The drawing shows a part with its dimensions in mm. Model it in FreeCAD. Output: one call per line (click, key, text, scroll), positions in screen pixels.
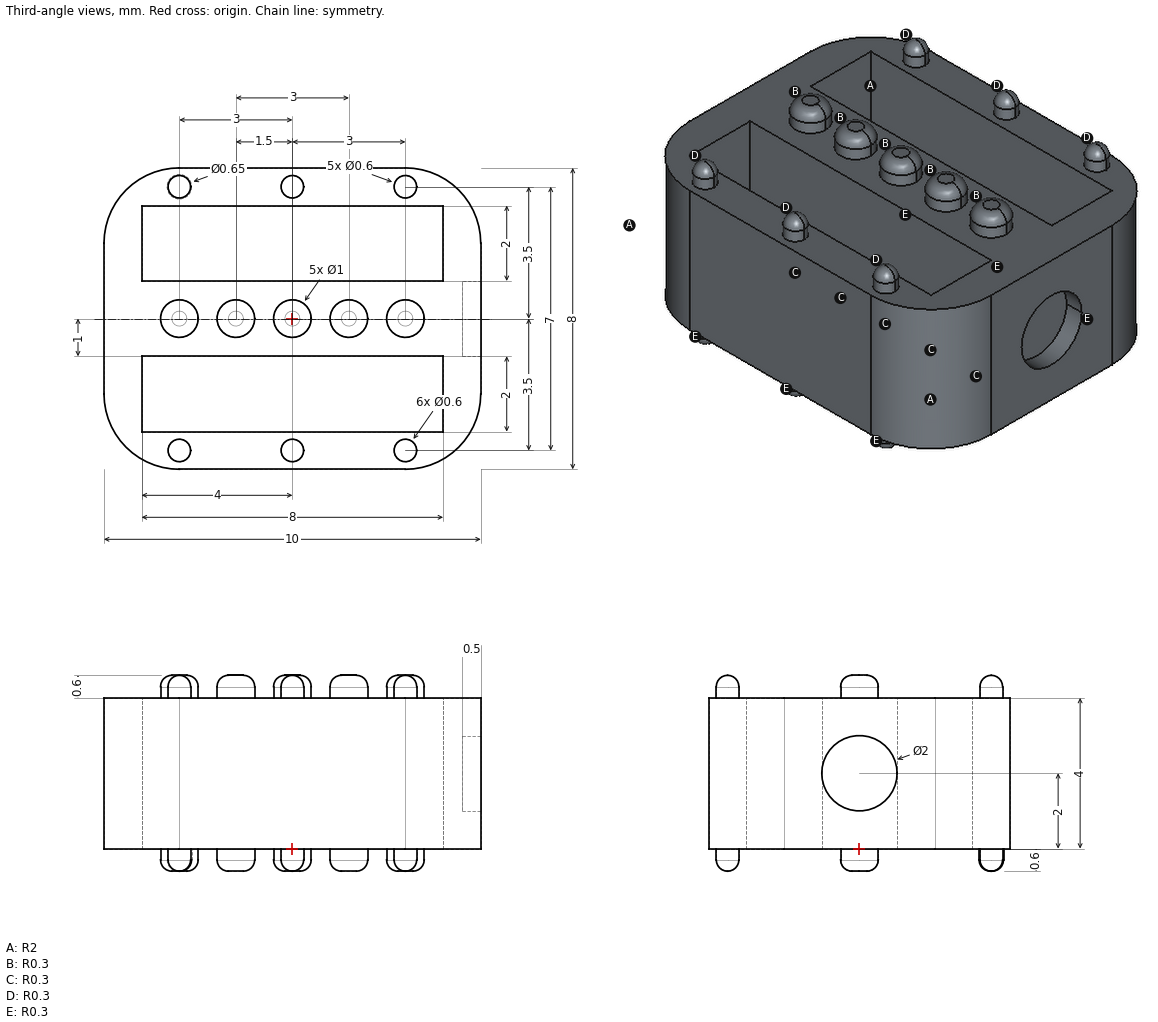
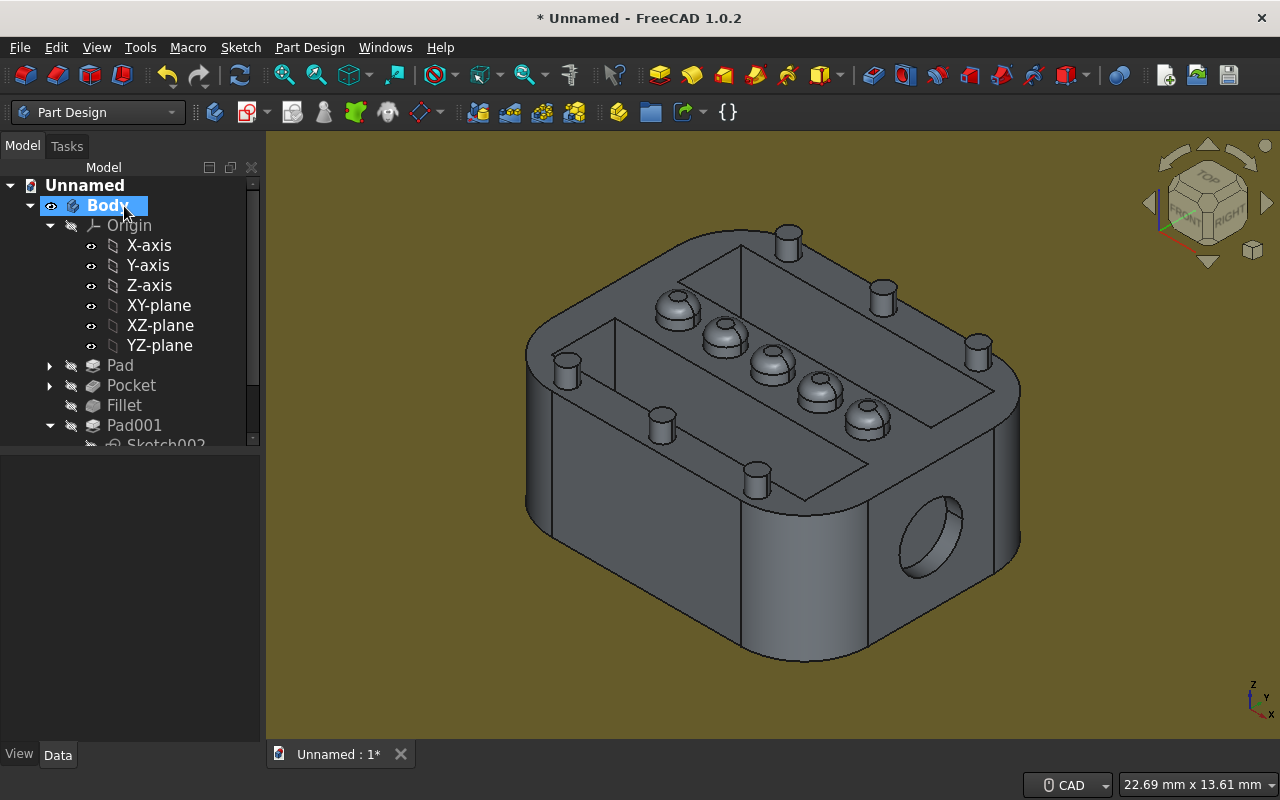
scroll(100, 321, down, 3)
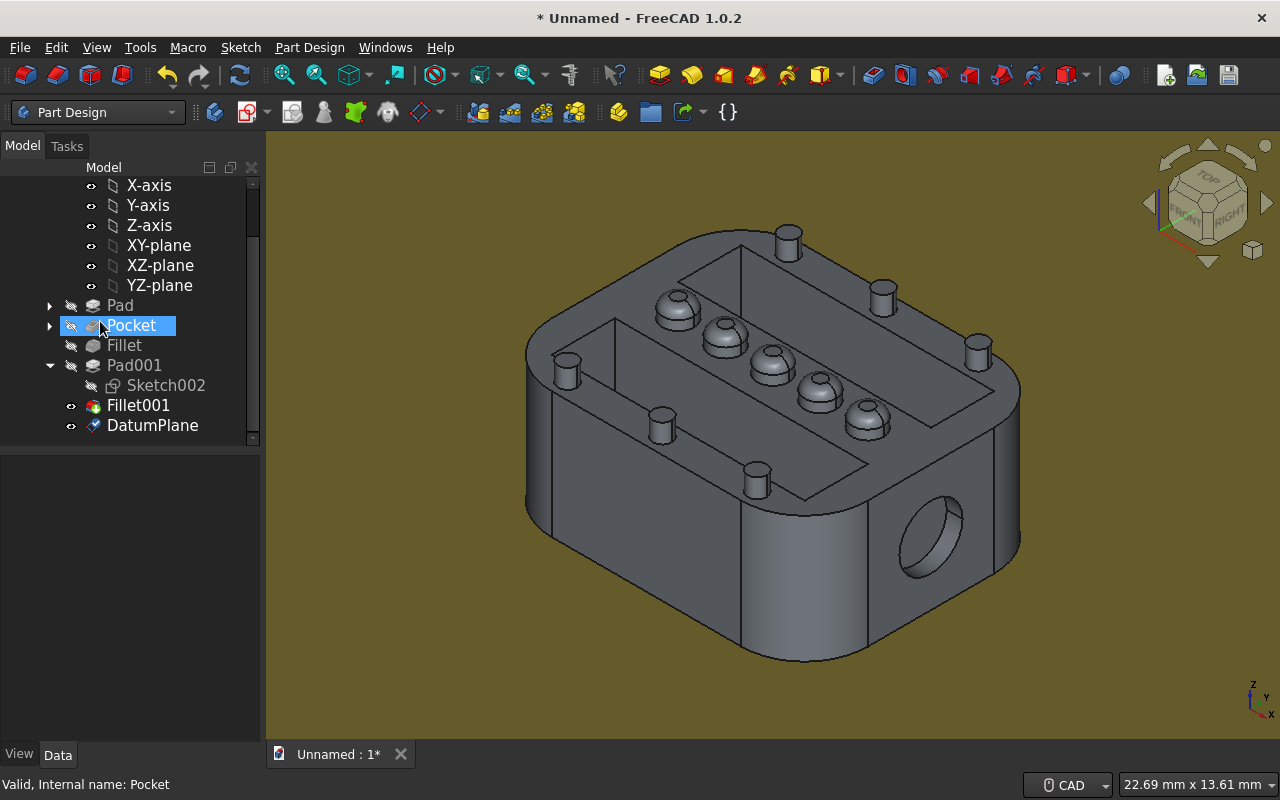
click(116, 426)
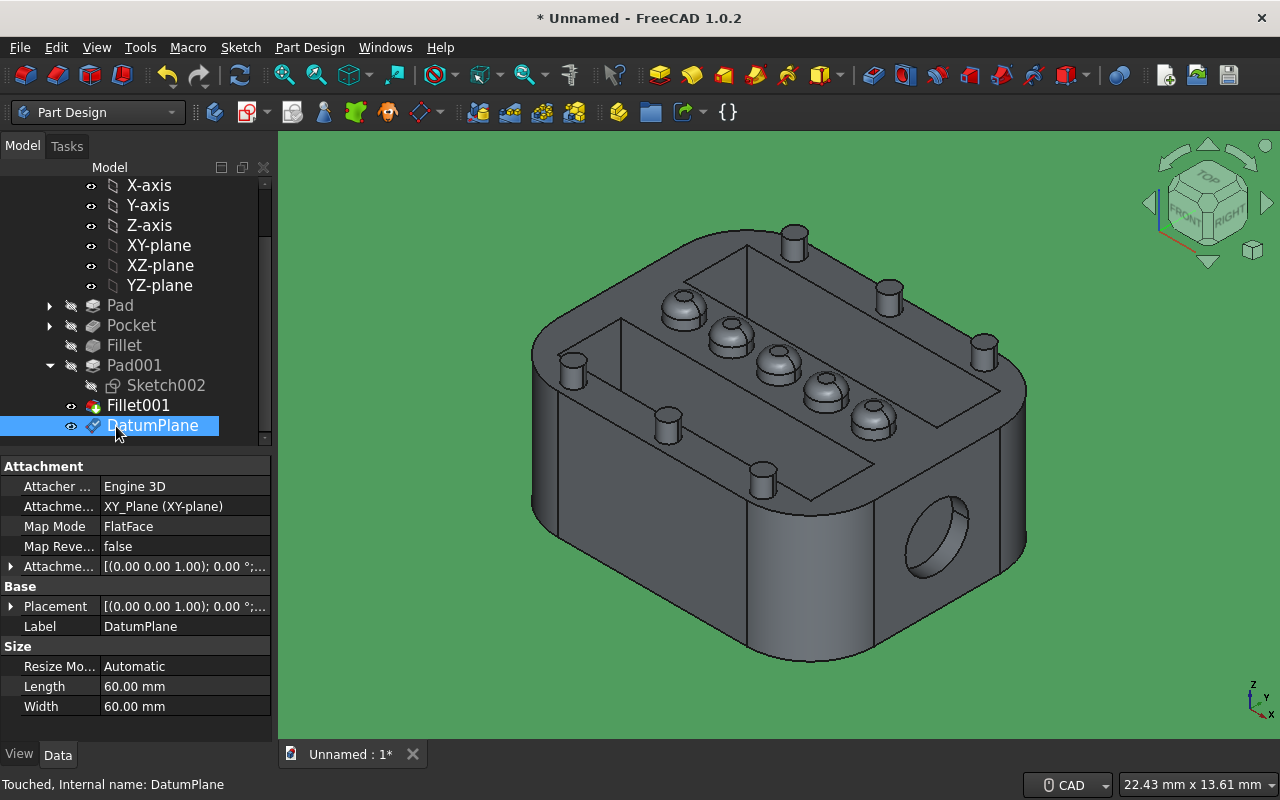
click(248, 112)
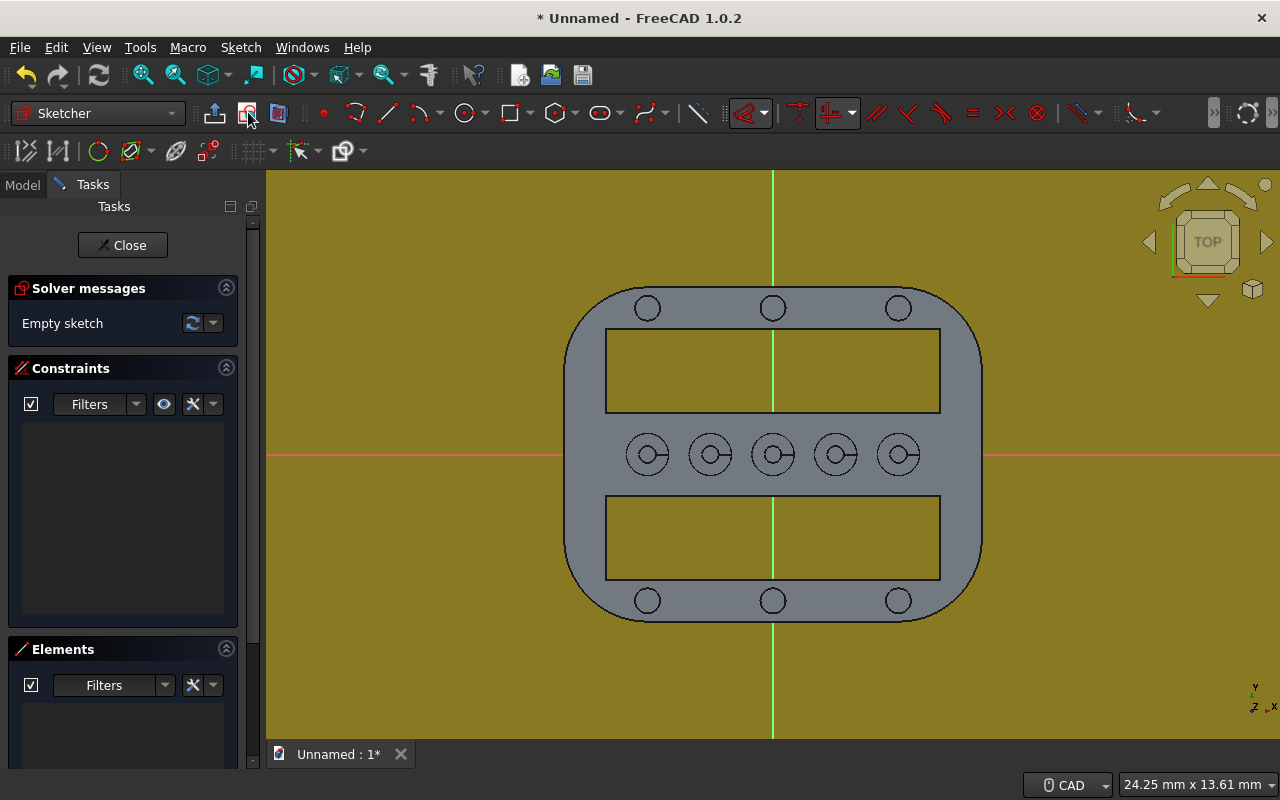
click(280, 114)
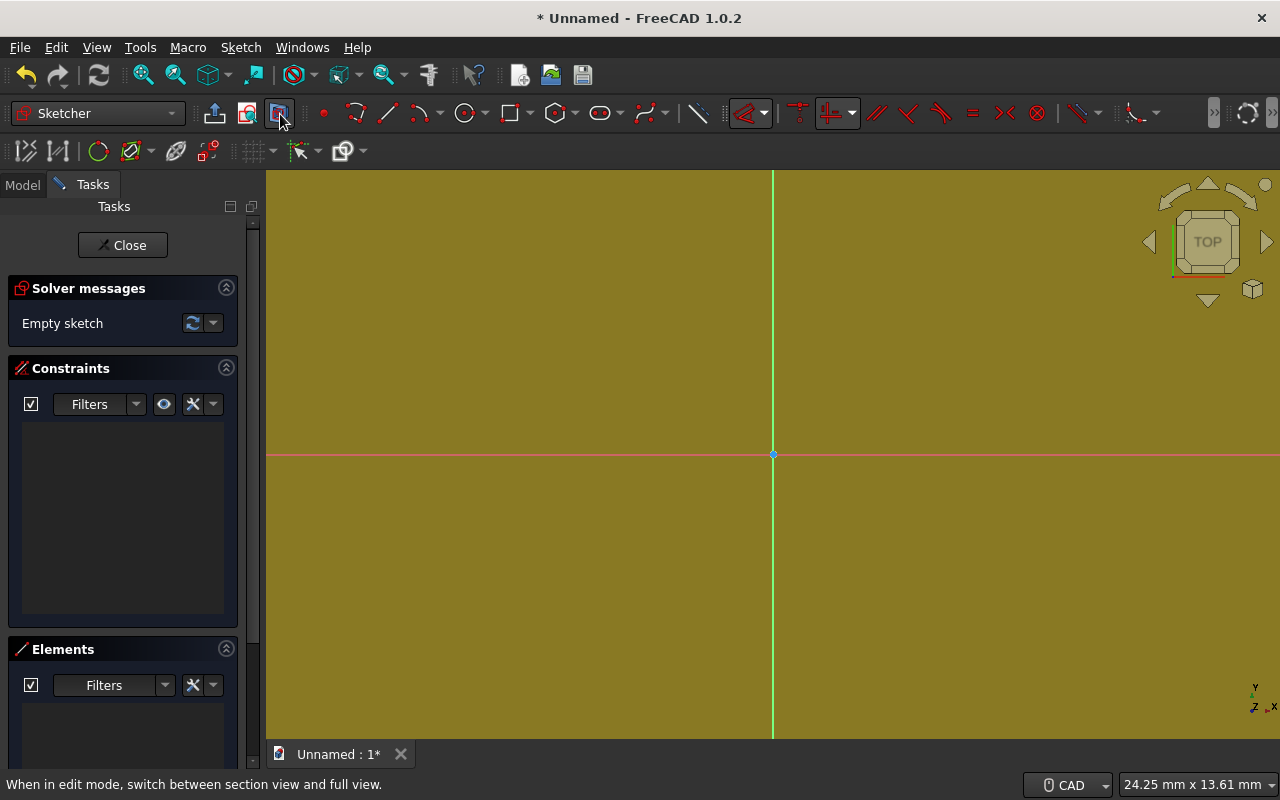
click(466, 114)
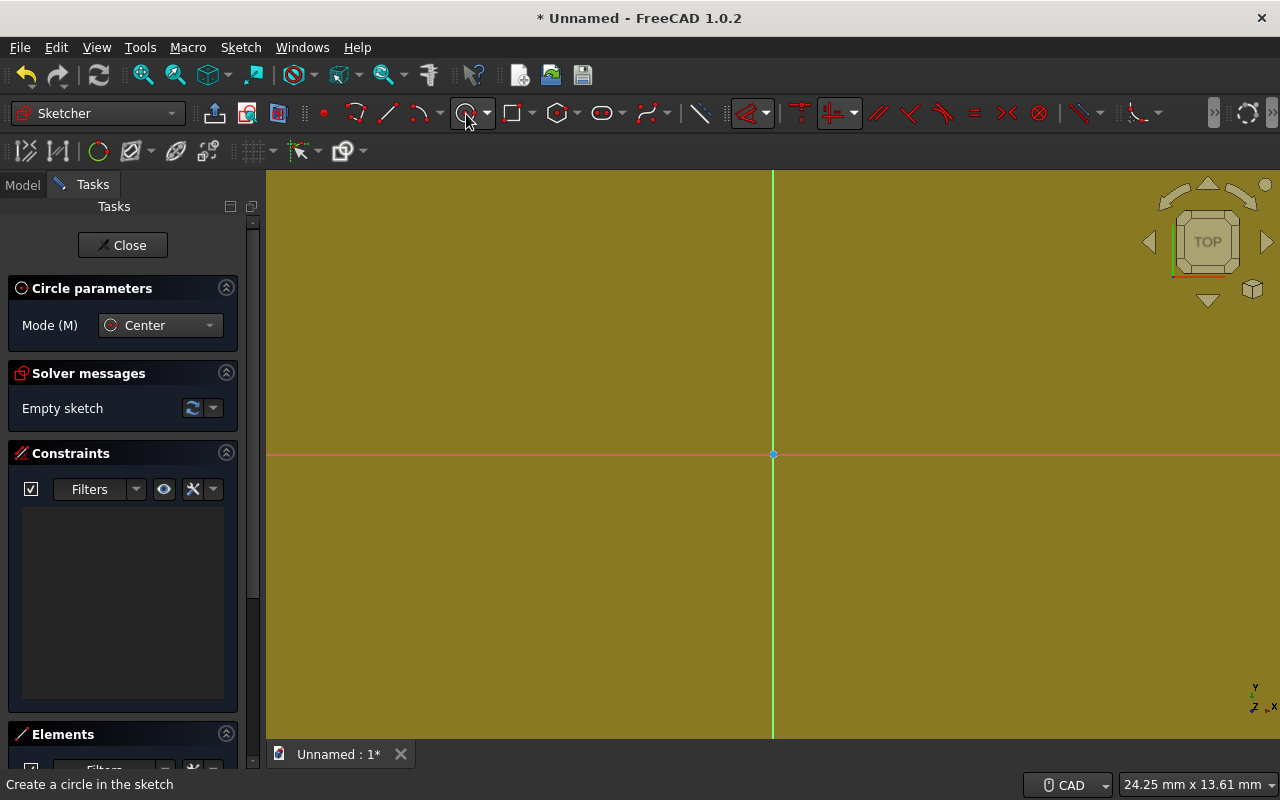
click(773, 454)
move(788, 440)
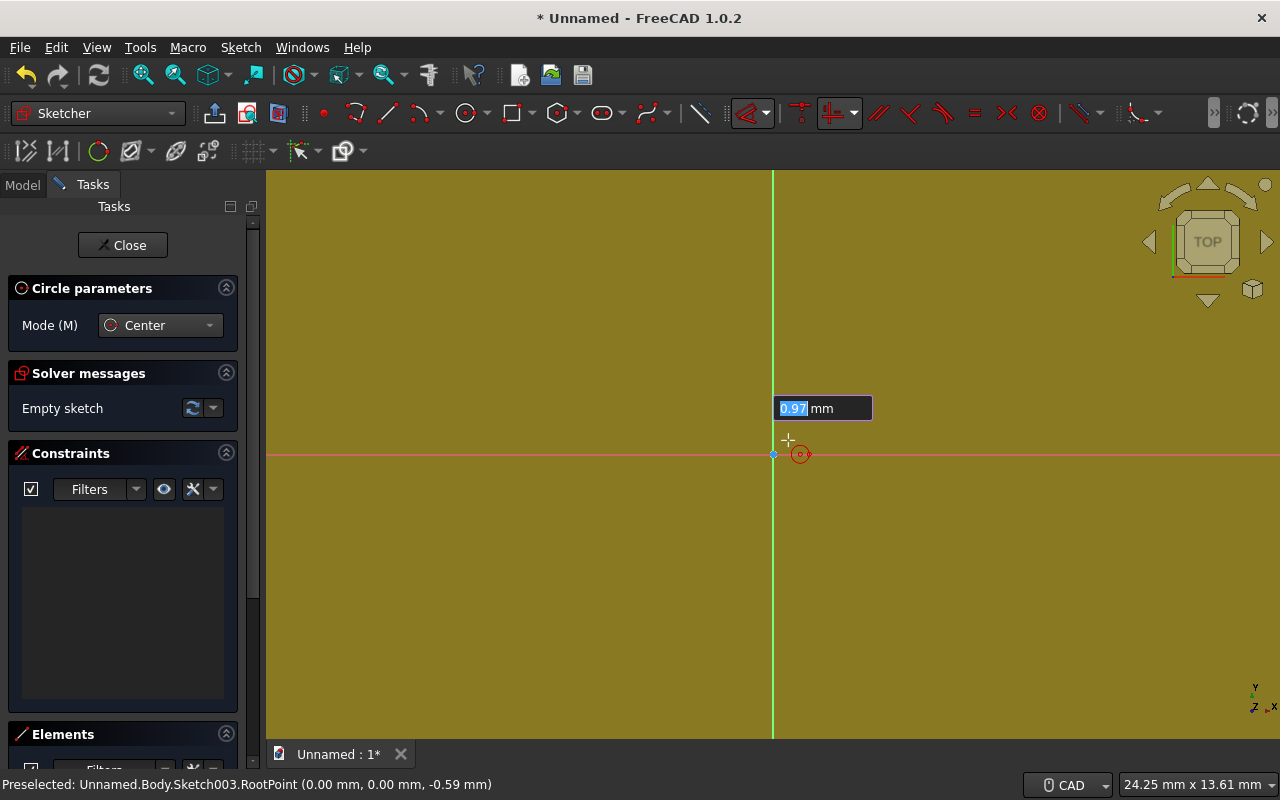
text(1)
key(Return)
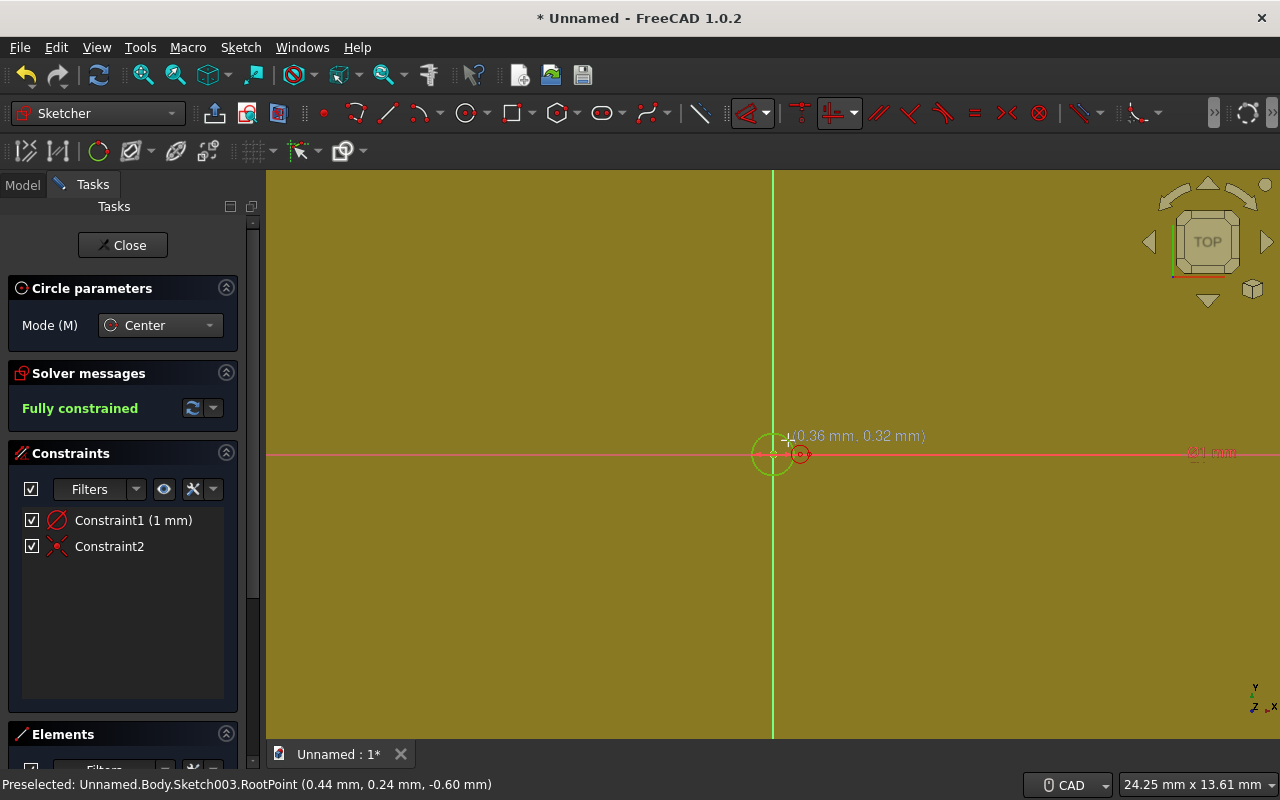
click(710, 454)
move(725, 440)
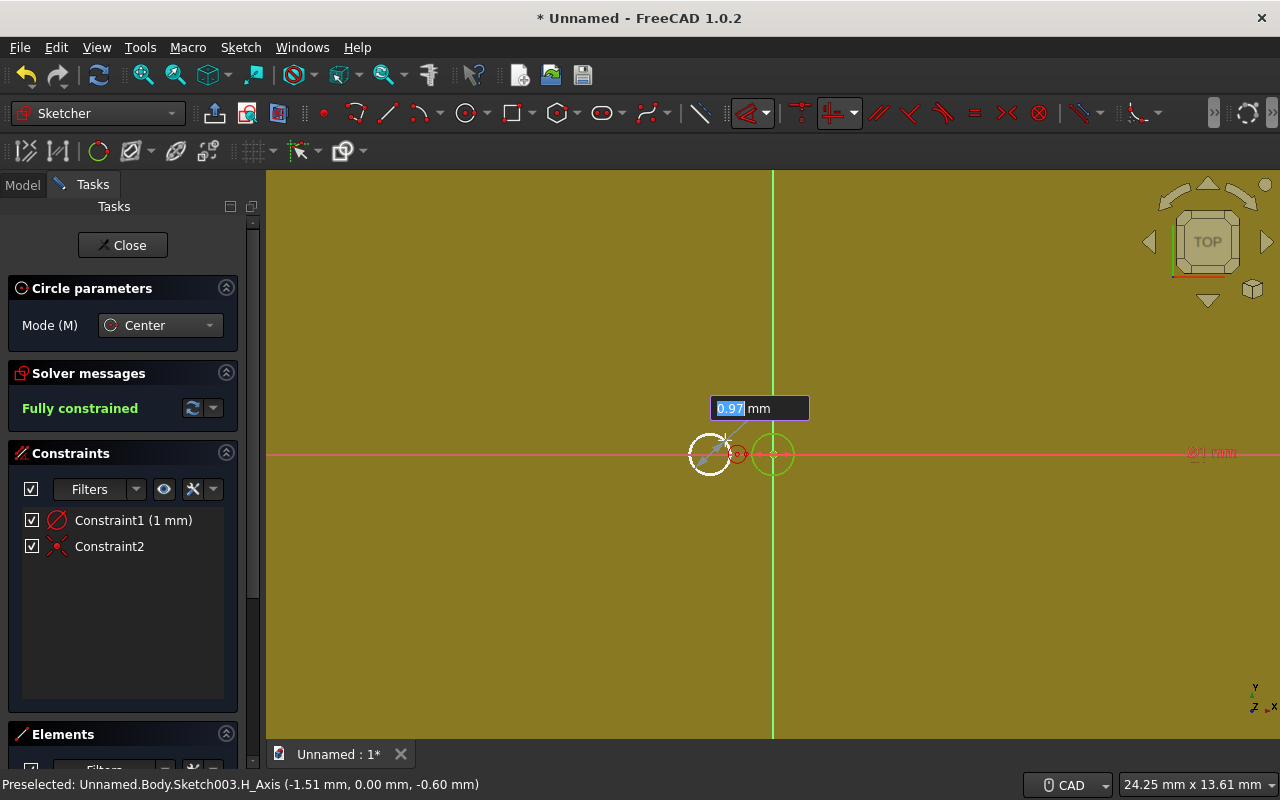
text(1)
key(Return)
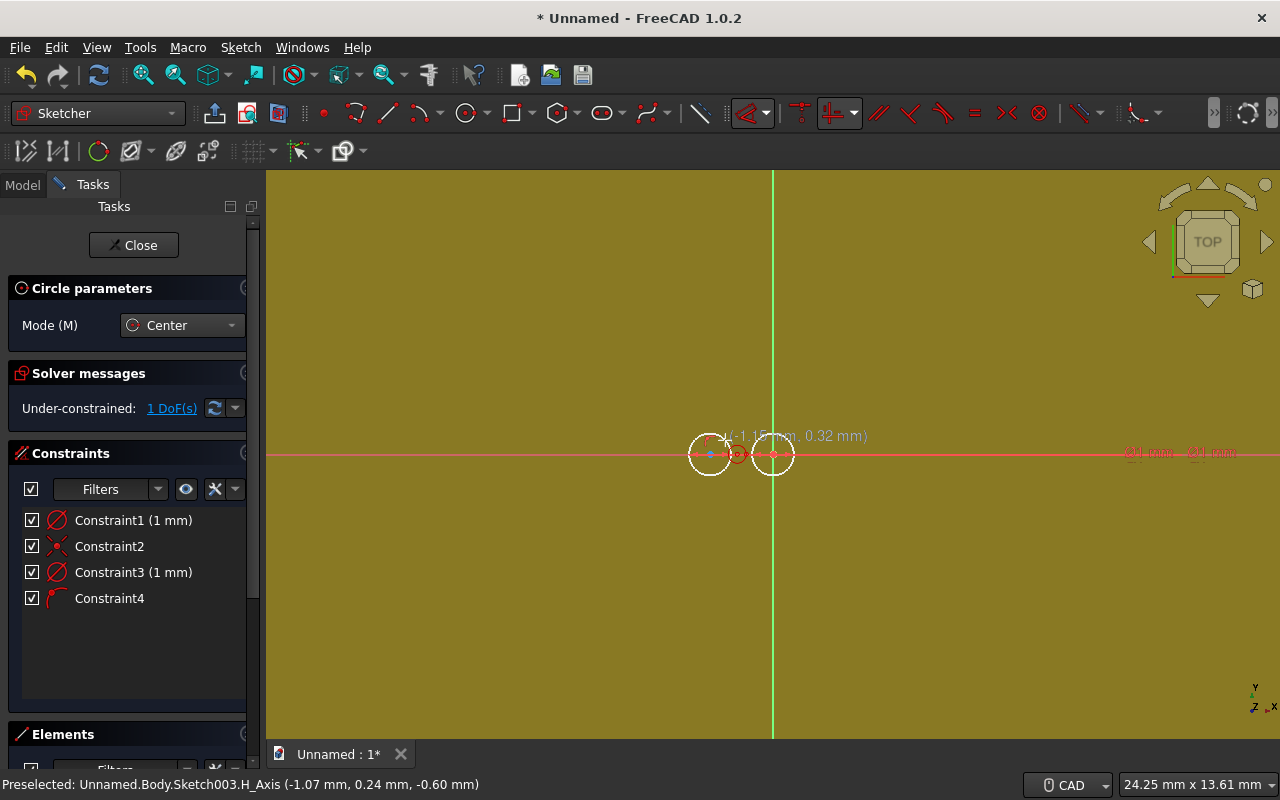
click(648, 454)
move(662, 440)